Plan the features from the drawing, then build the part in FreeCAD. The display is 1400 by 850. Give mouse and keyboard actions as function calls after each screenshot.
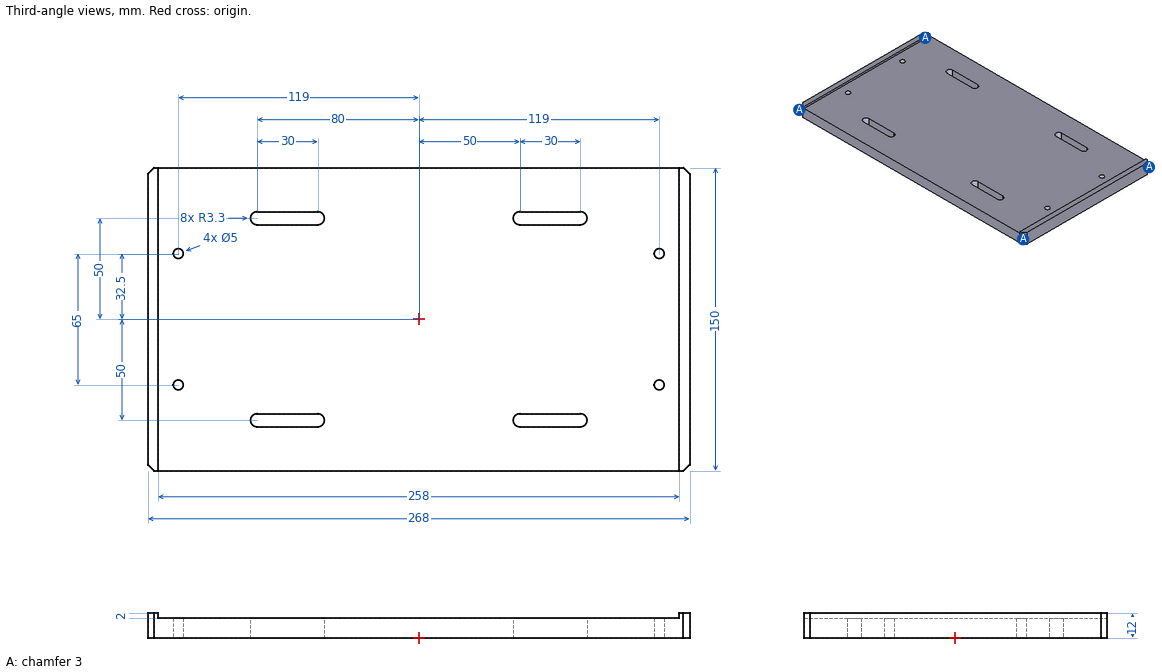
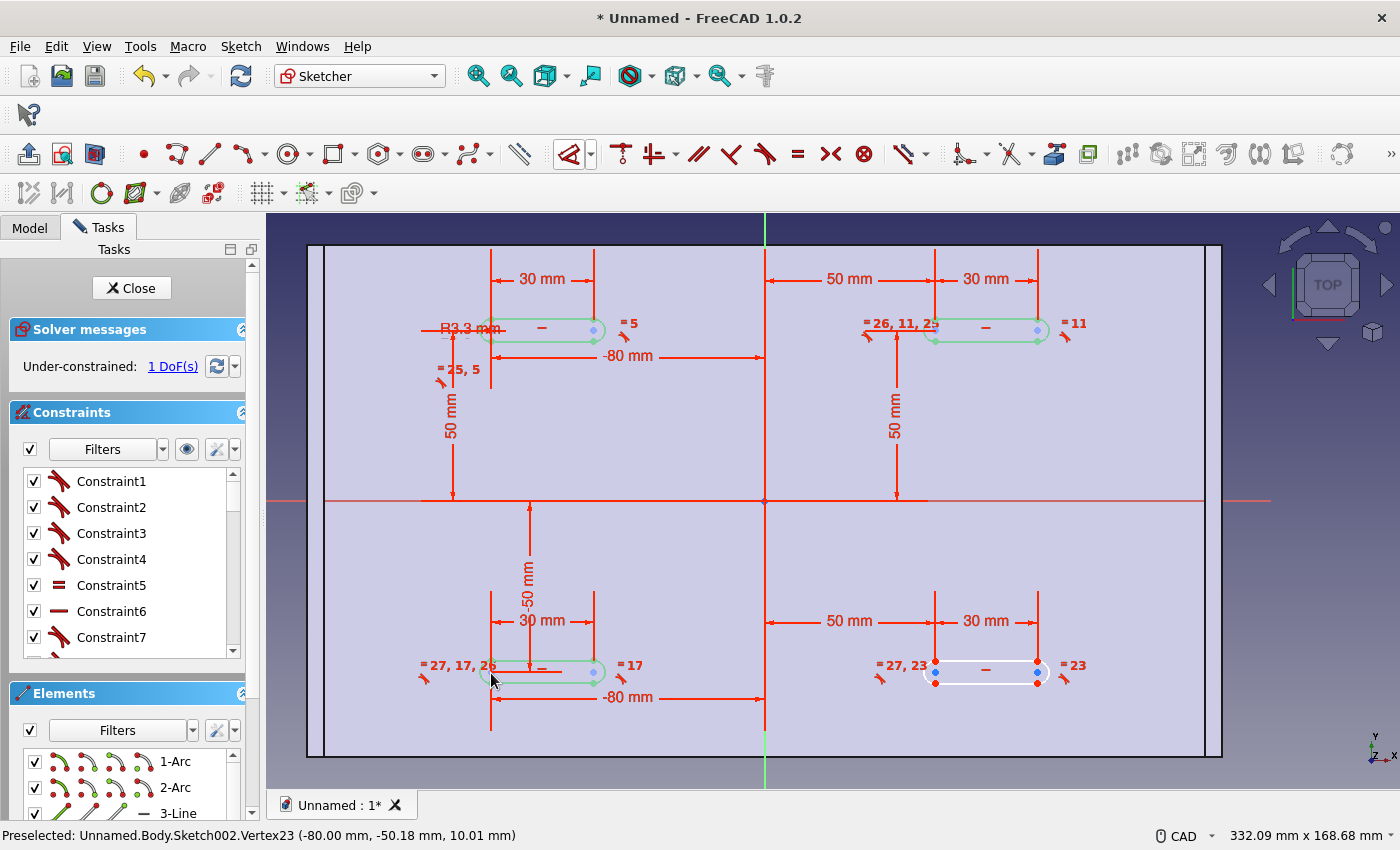
click(935, 673)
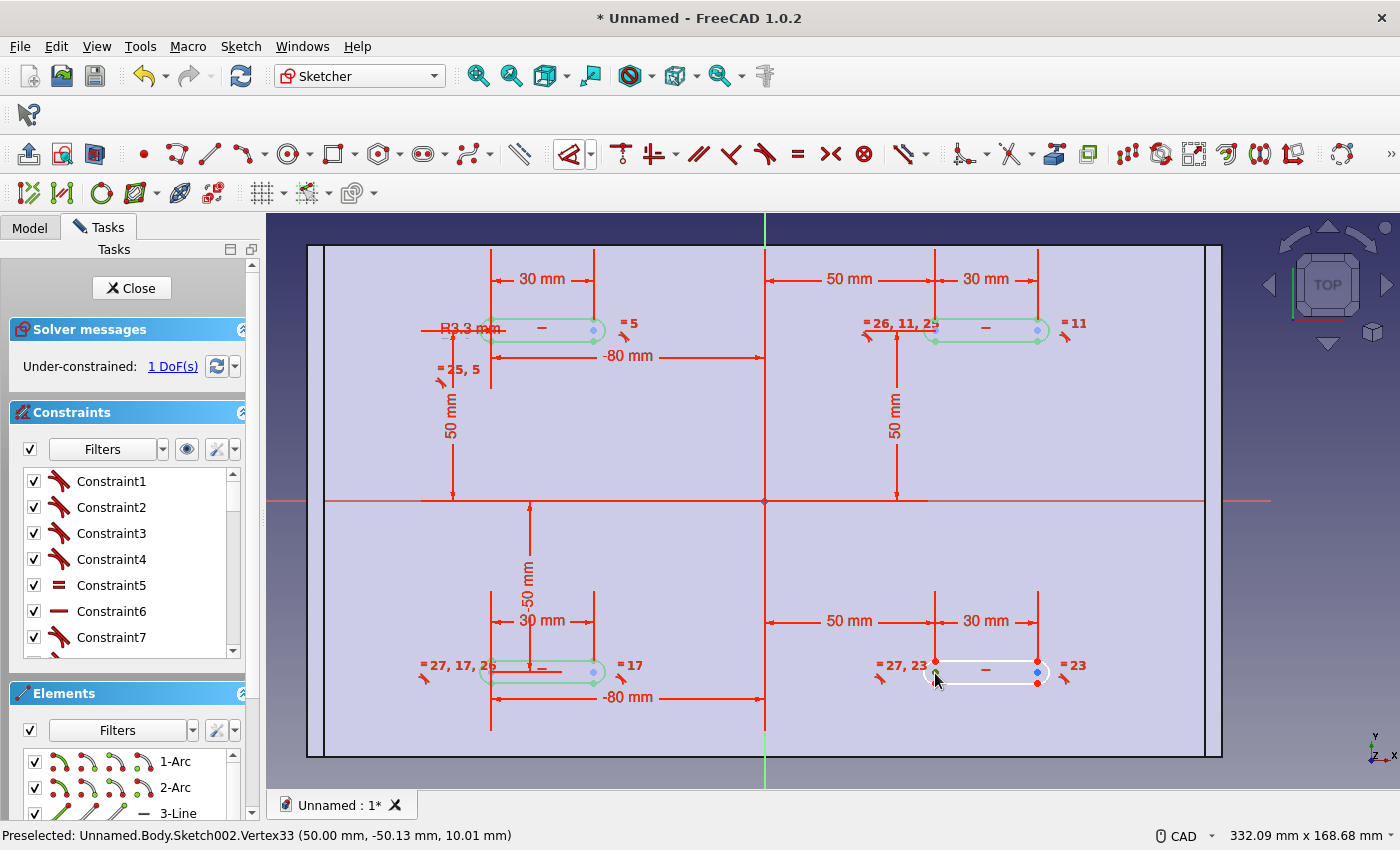
key(i)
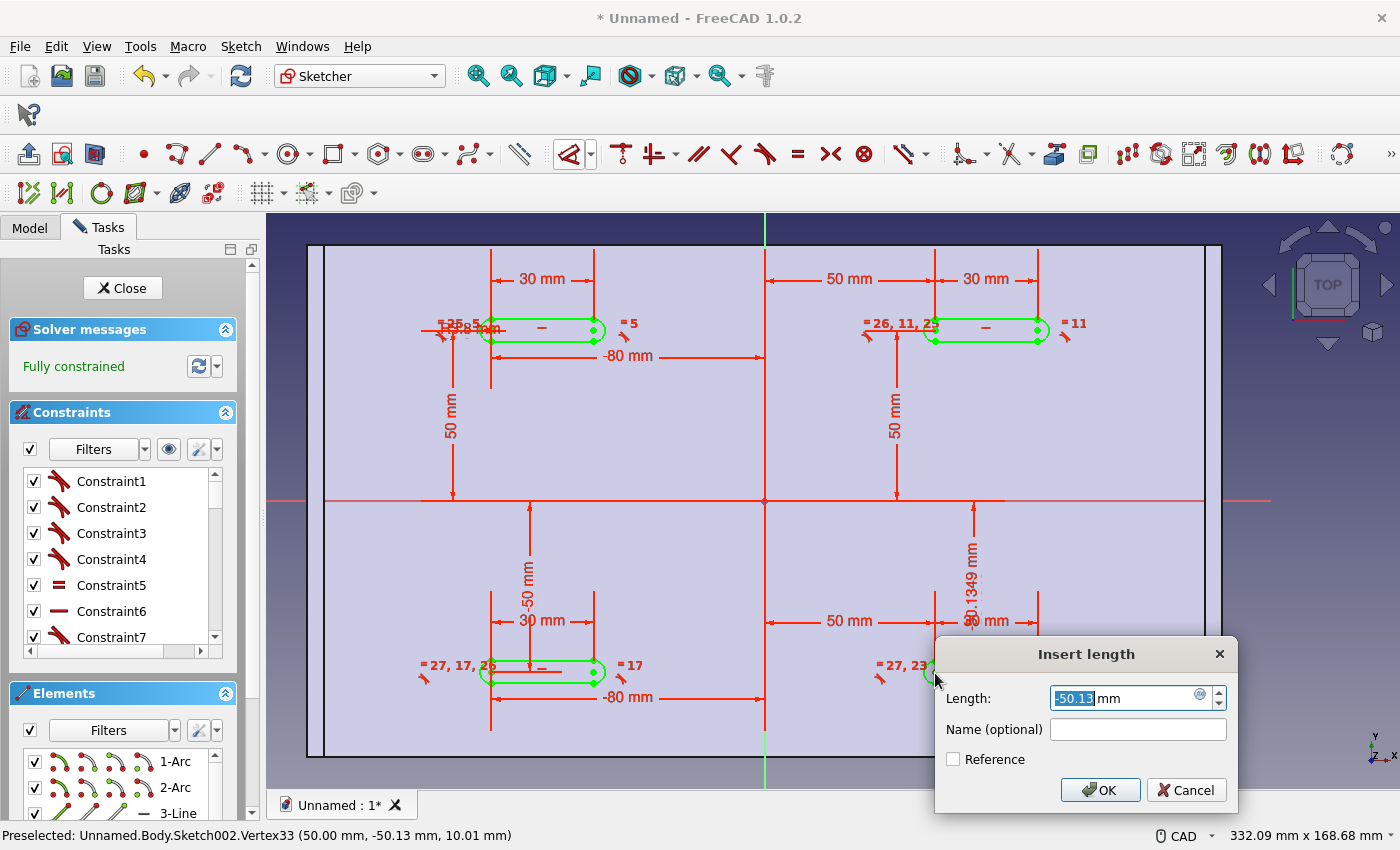
text(-50)
key(Return)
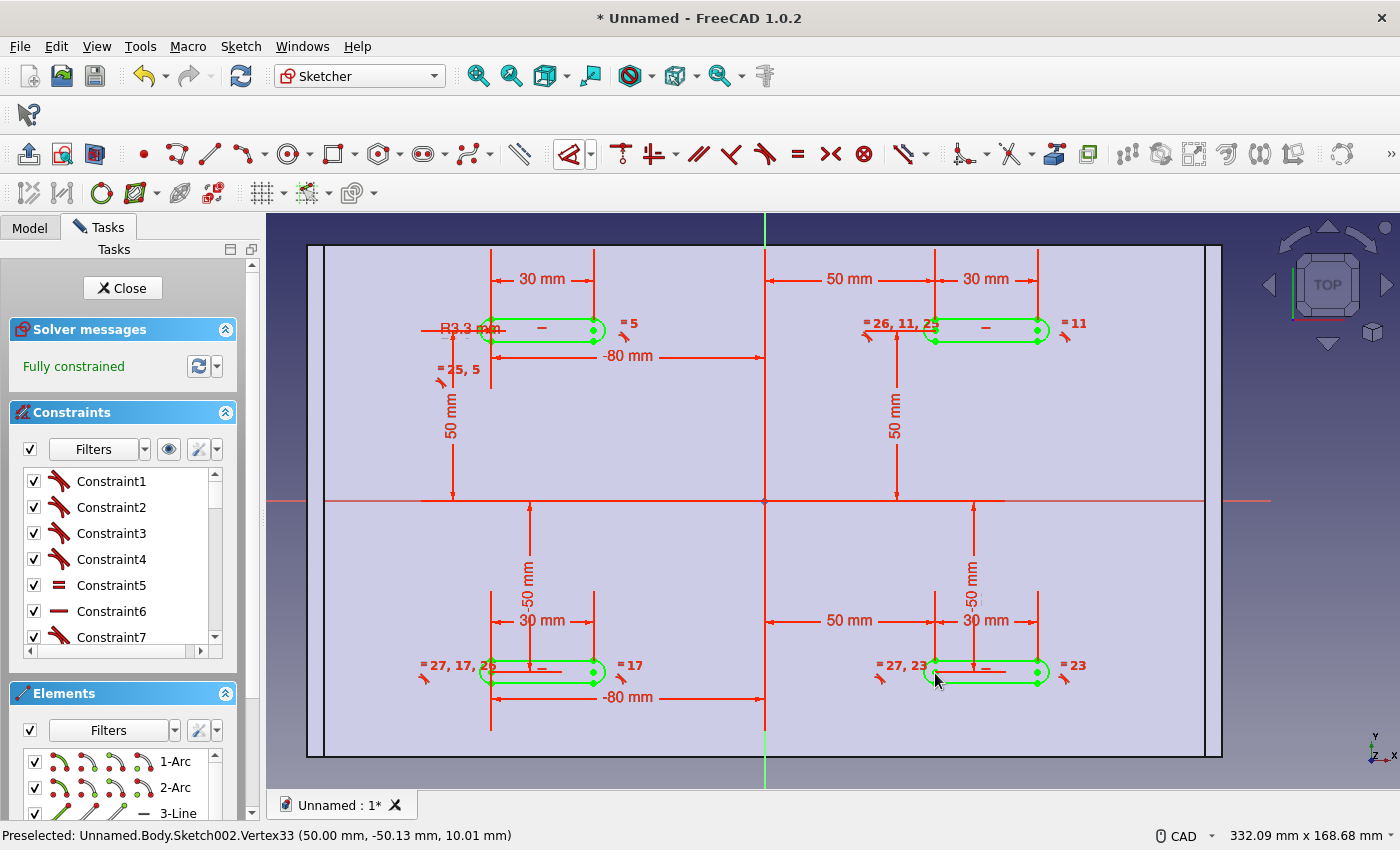
click(123, 288)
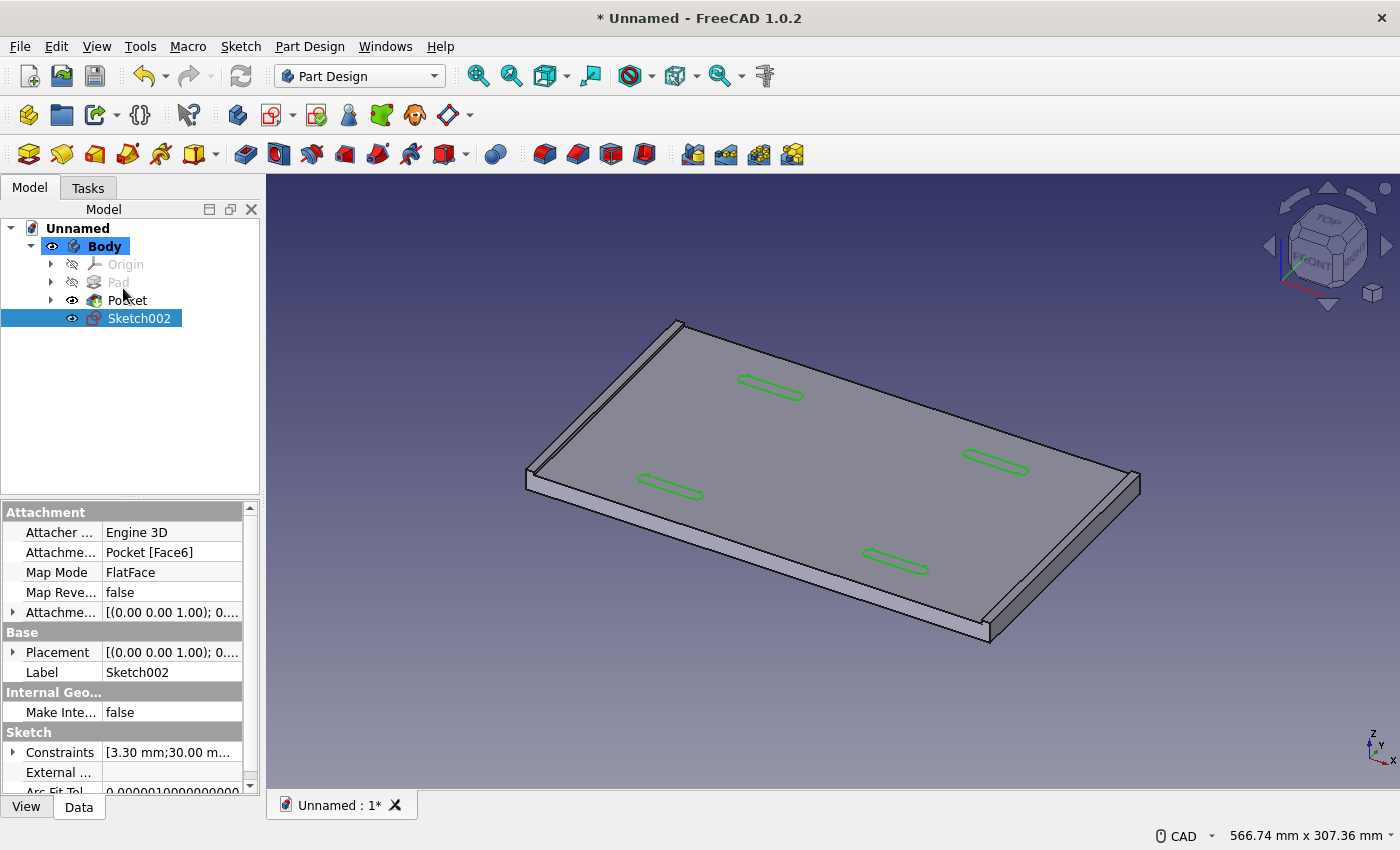
click(246, 154)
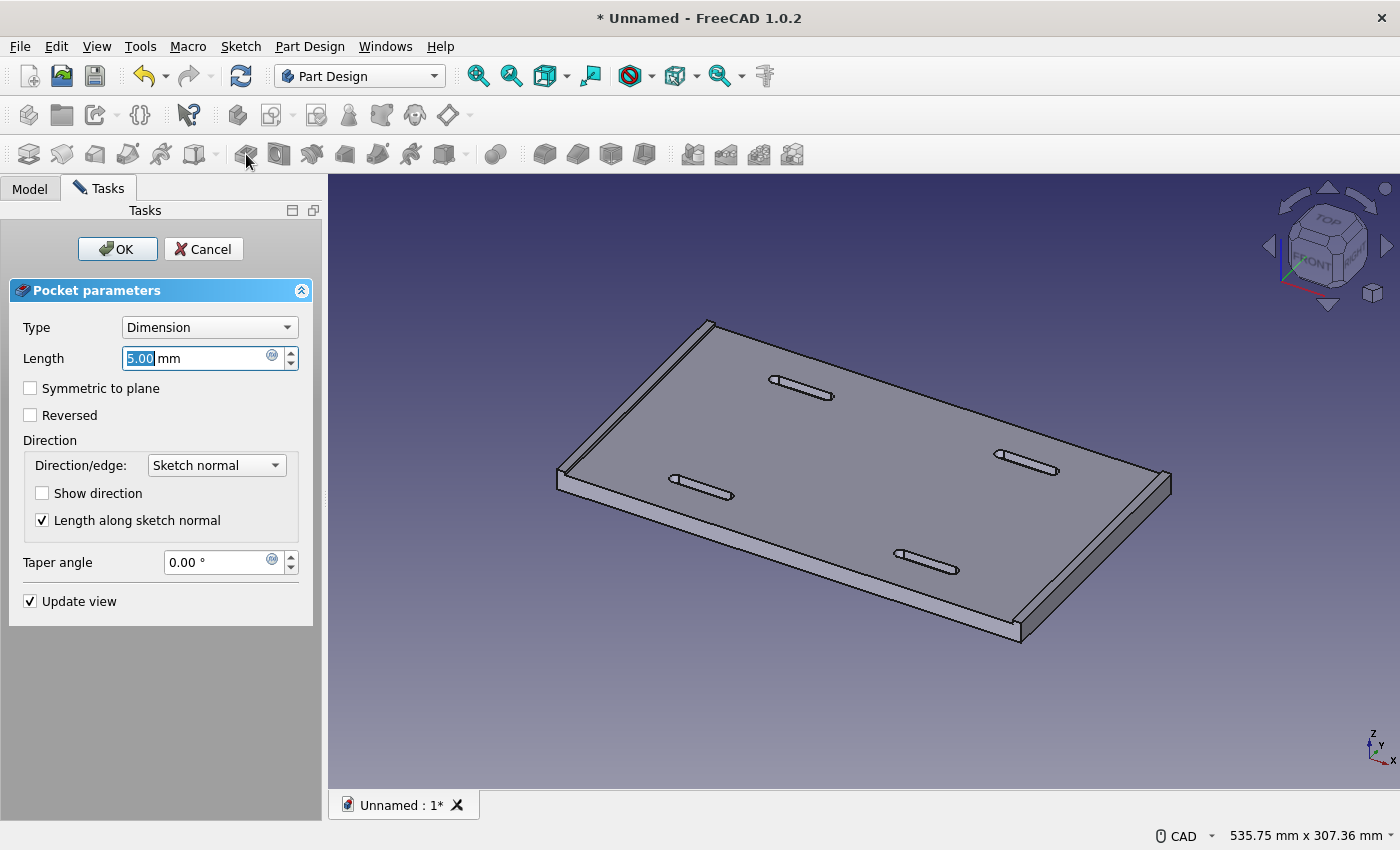
click(210, 328)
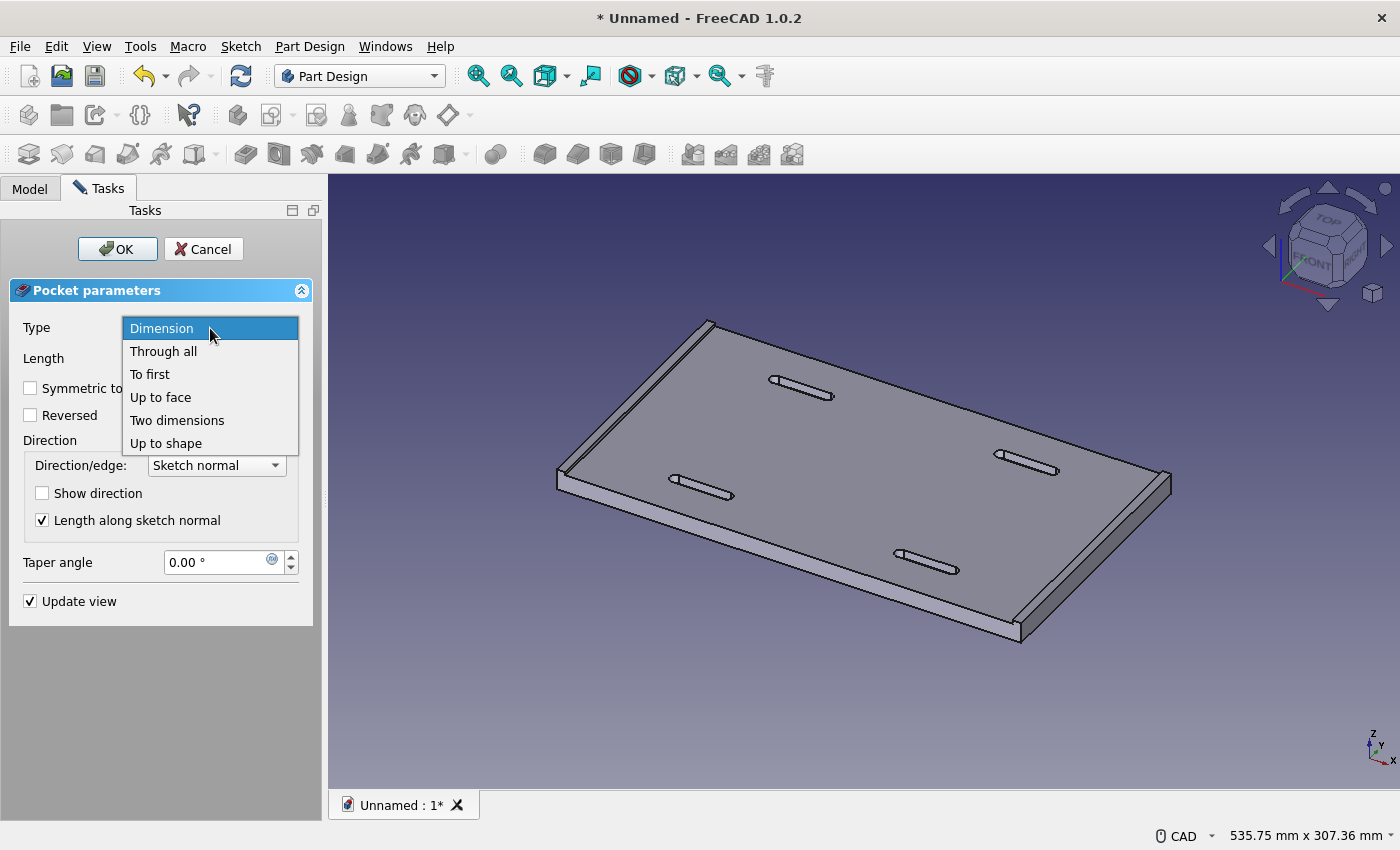
click(208, 352)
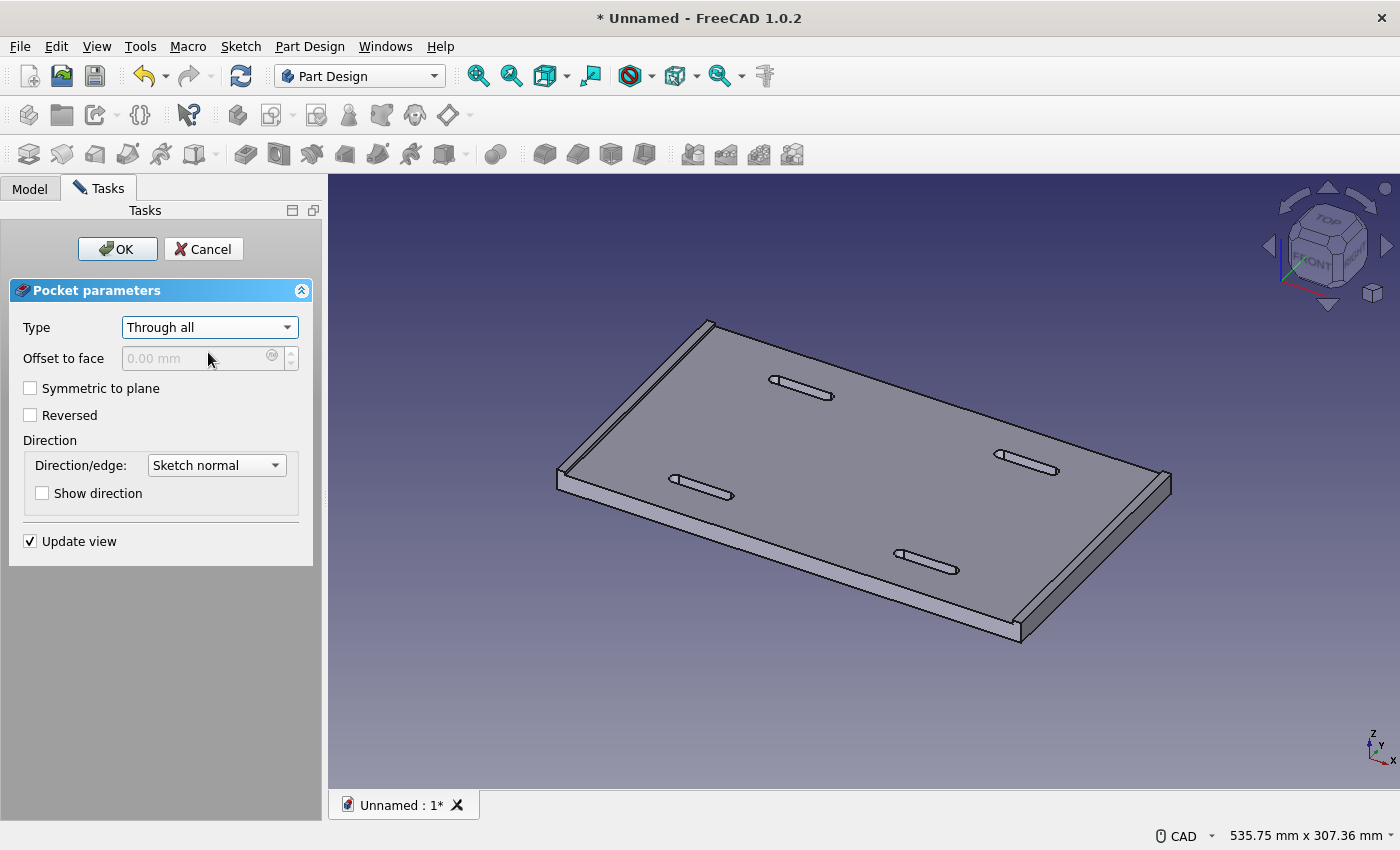
click(118, 249)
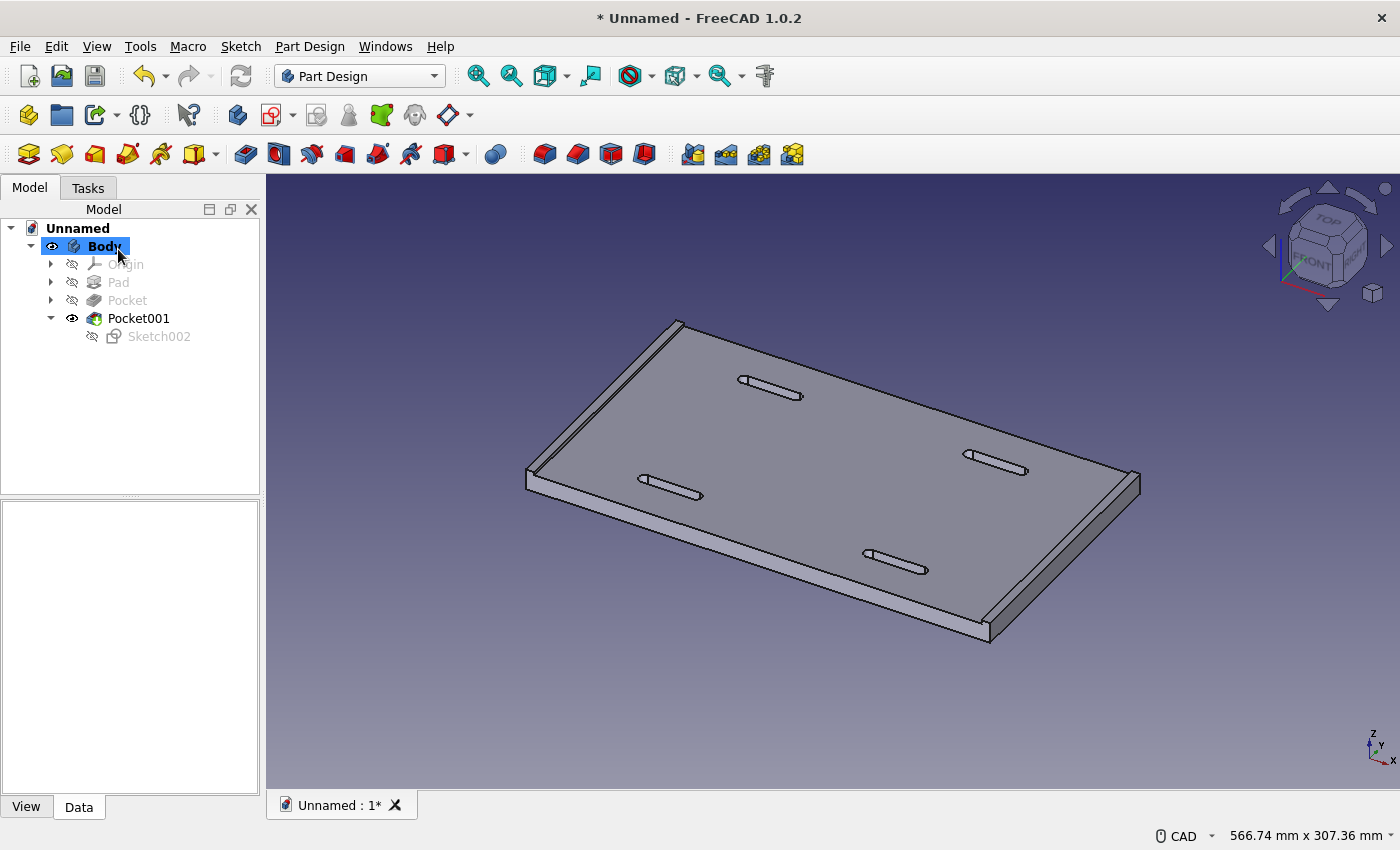
click(833, 474)